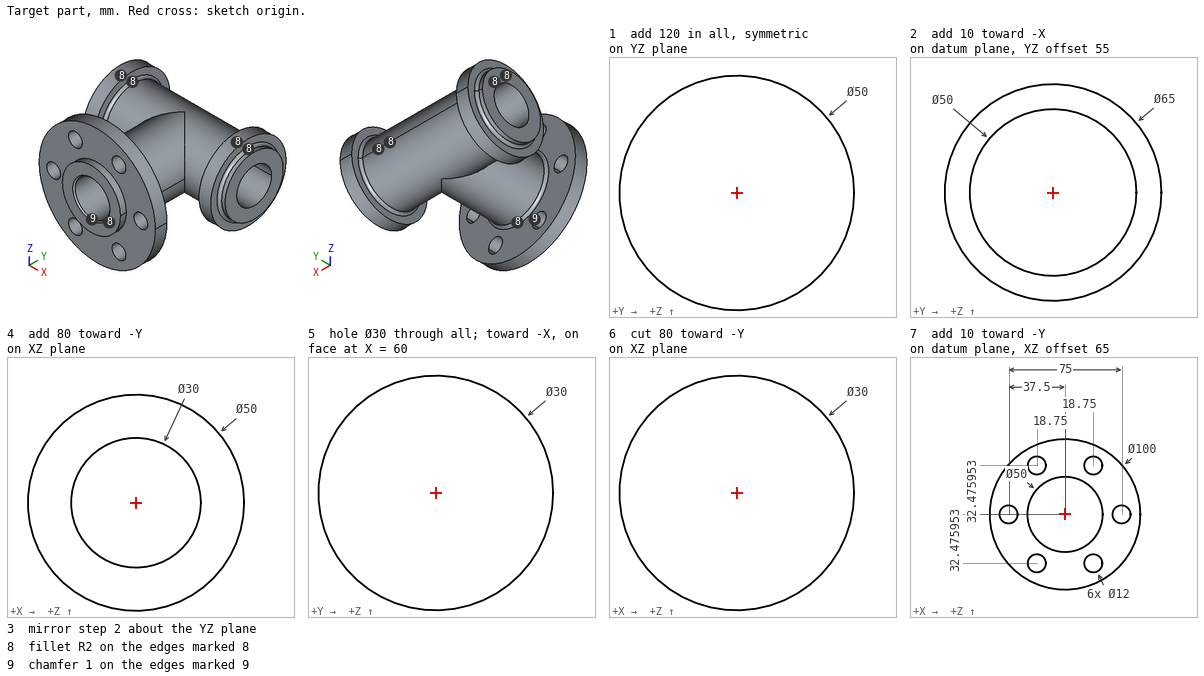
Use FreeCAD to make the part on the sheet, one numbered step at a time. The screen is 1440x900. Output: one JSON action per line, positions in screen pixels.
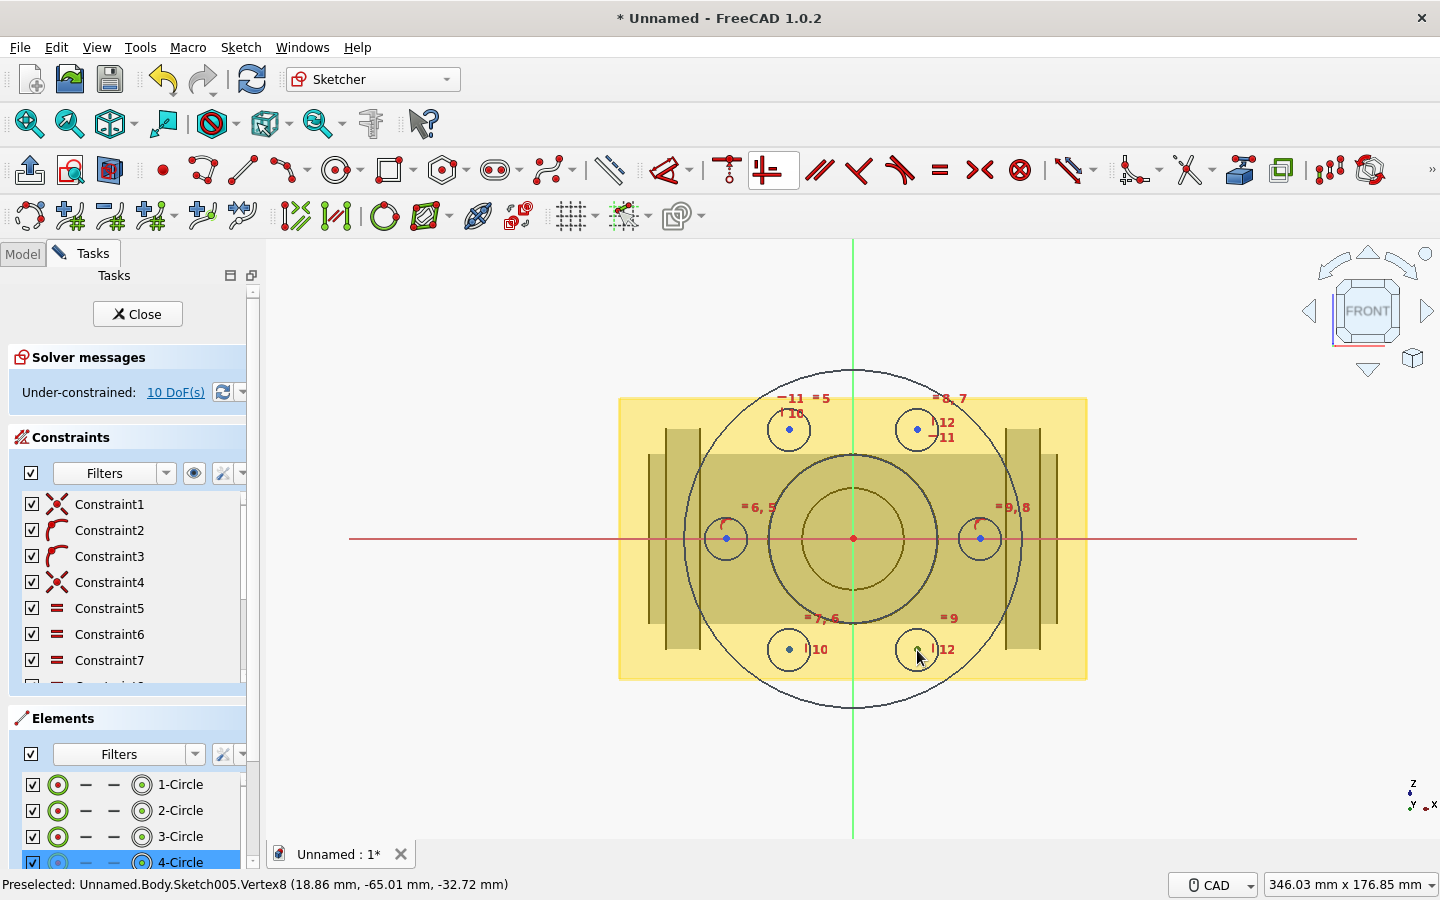
{"action": "key", "text": "h"}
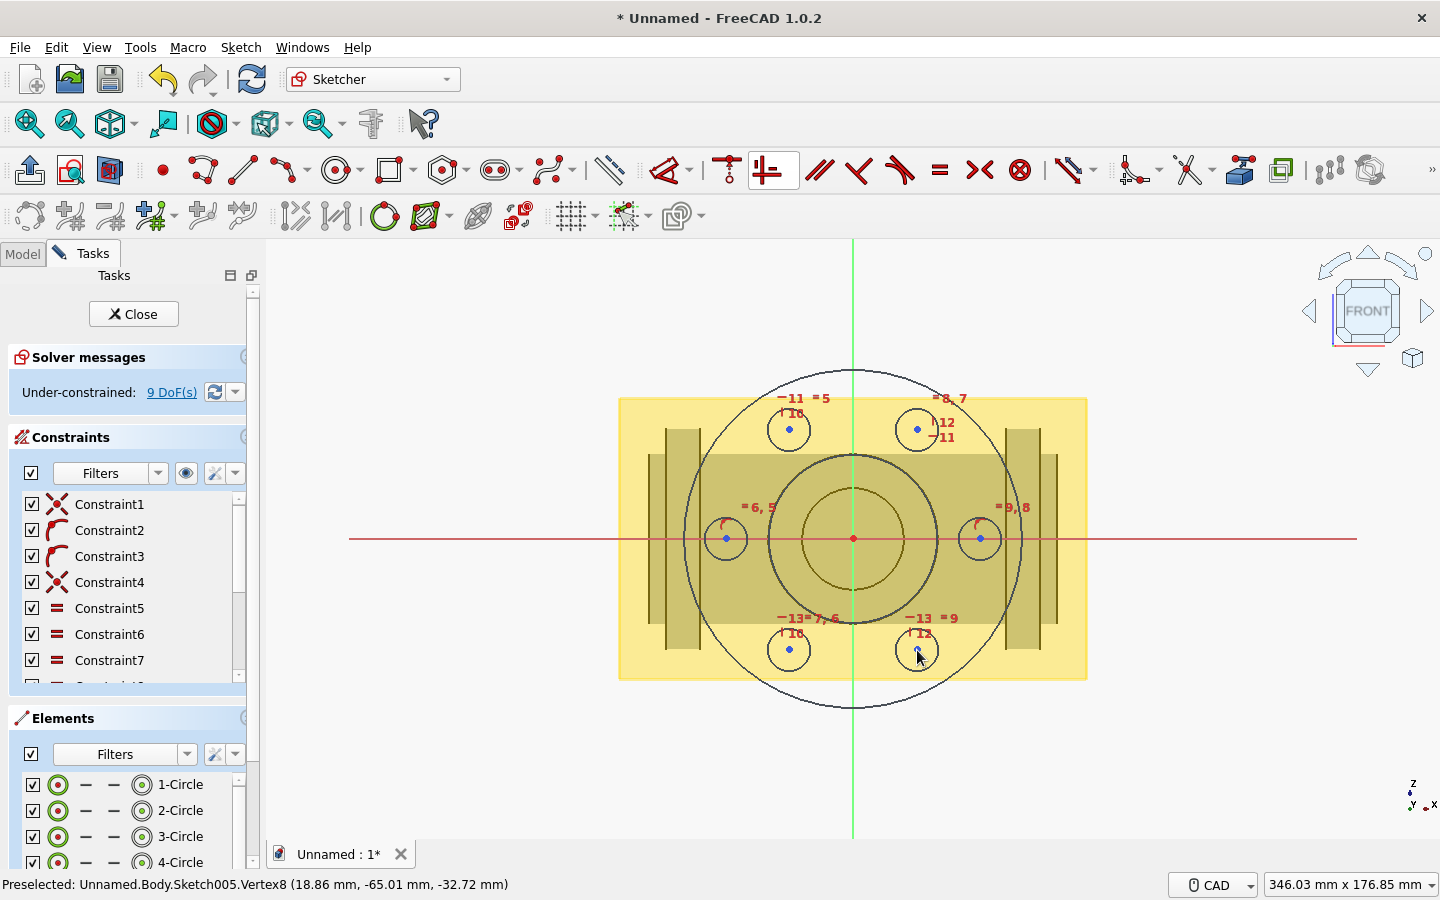
{"action": "left_click", "coordinate": [972, 419]}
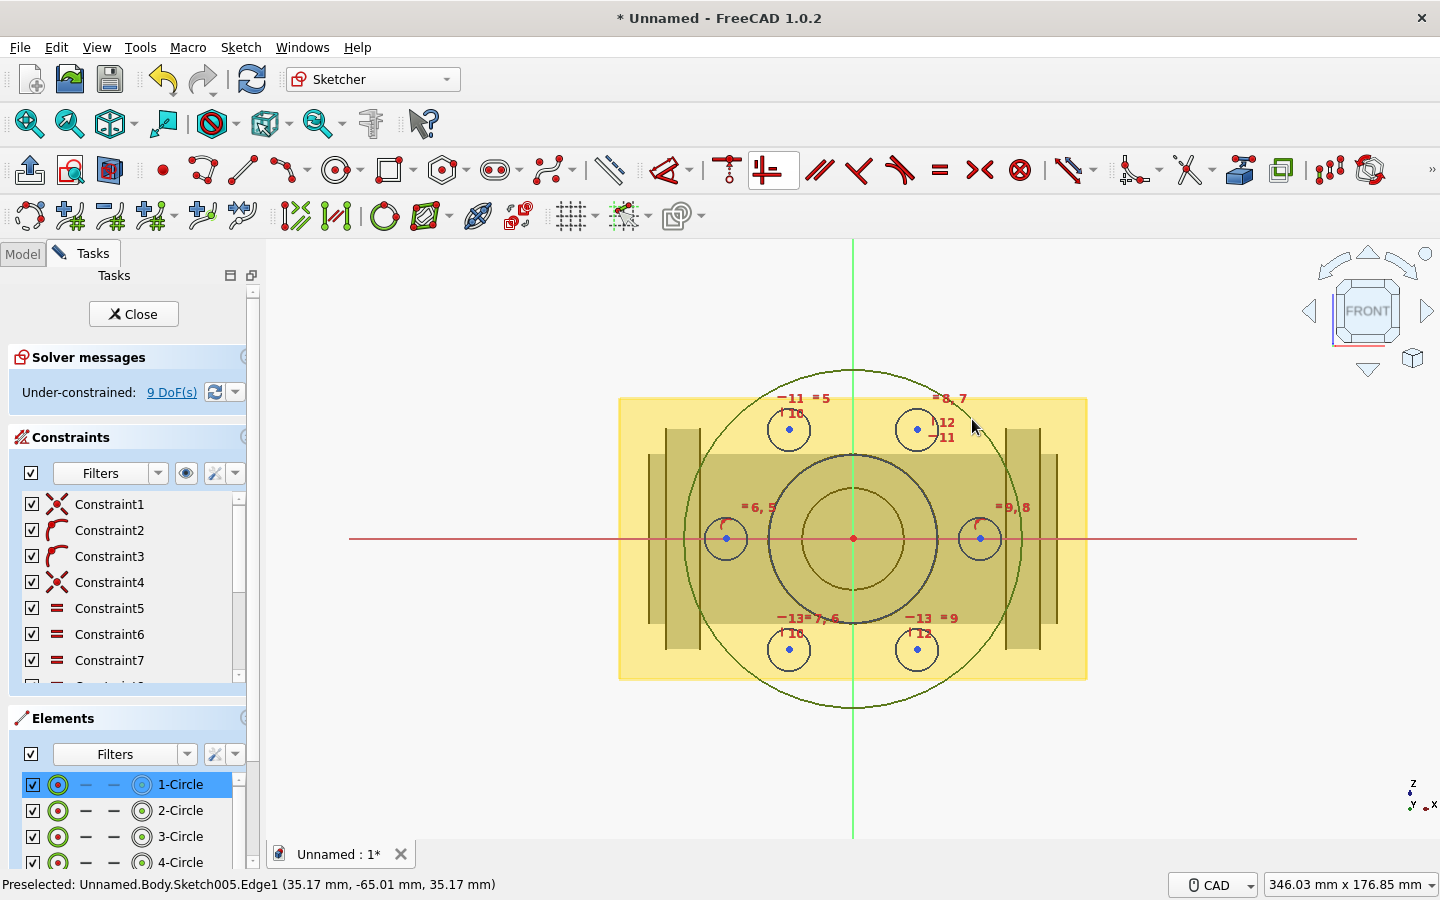
{"action": "key", "text": "k o"}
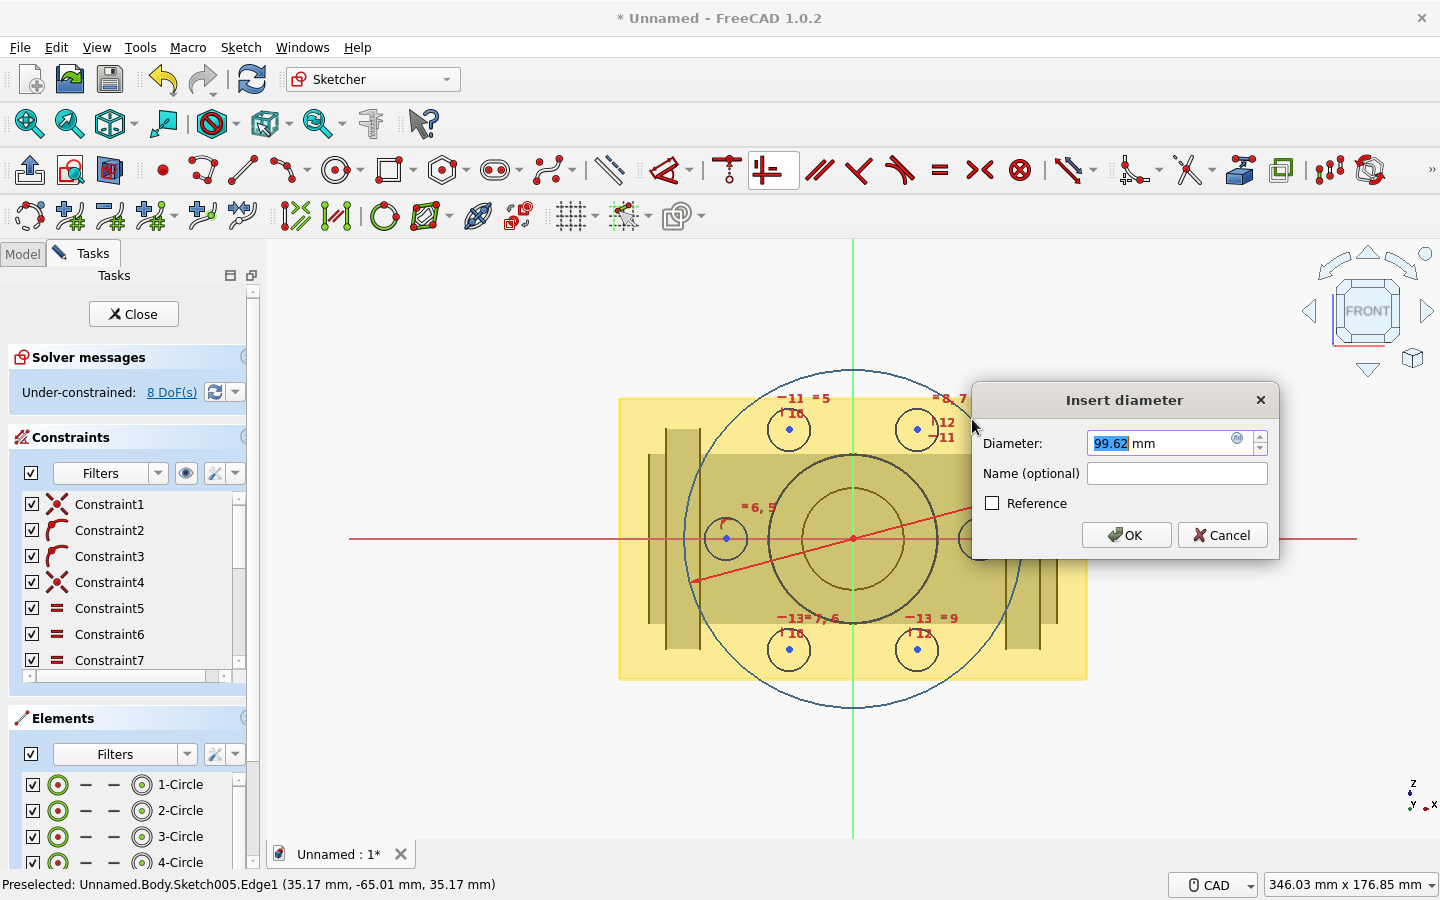
{"action": "type", "text": "100"}
{"action": "key", "text": "Return"}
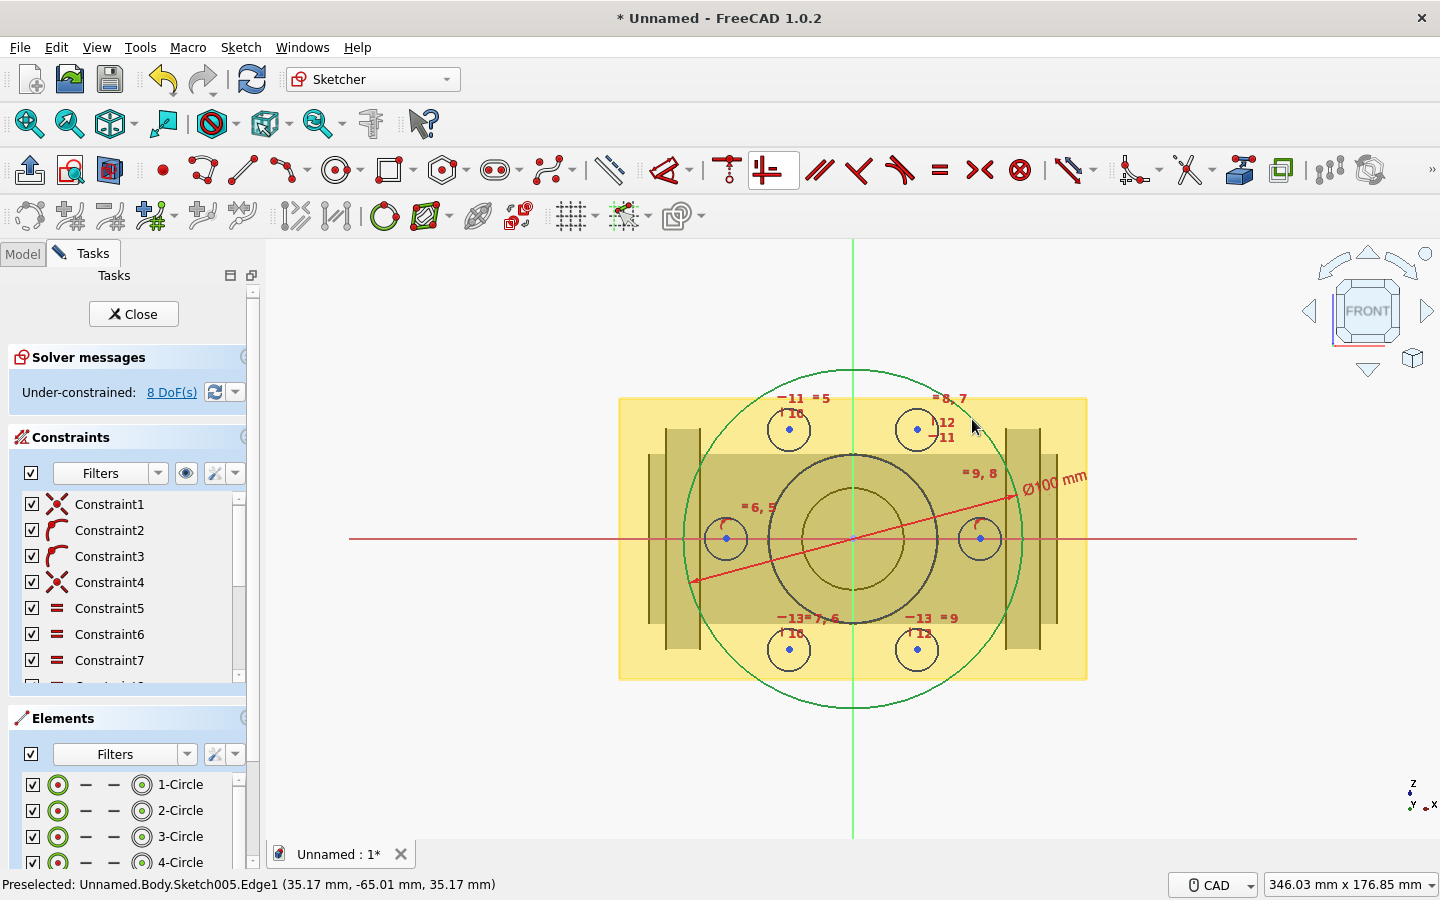
{"action": "left_click", "coordinate": [804, 415]}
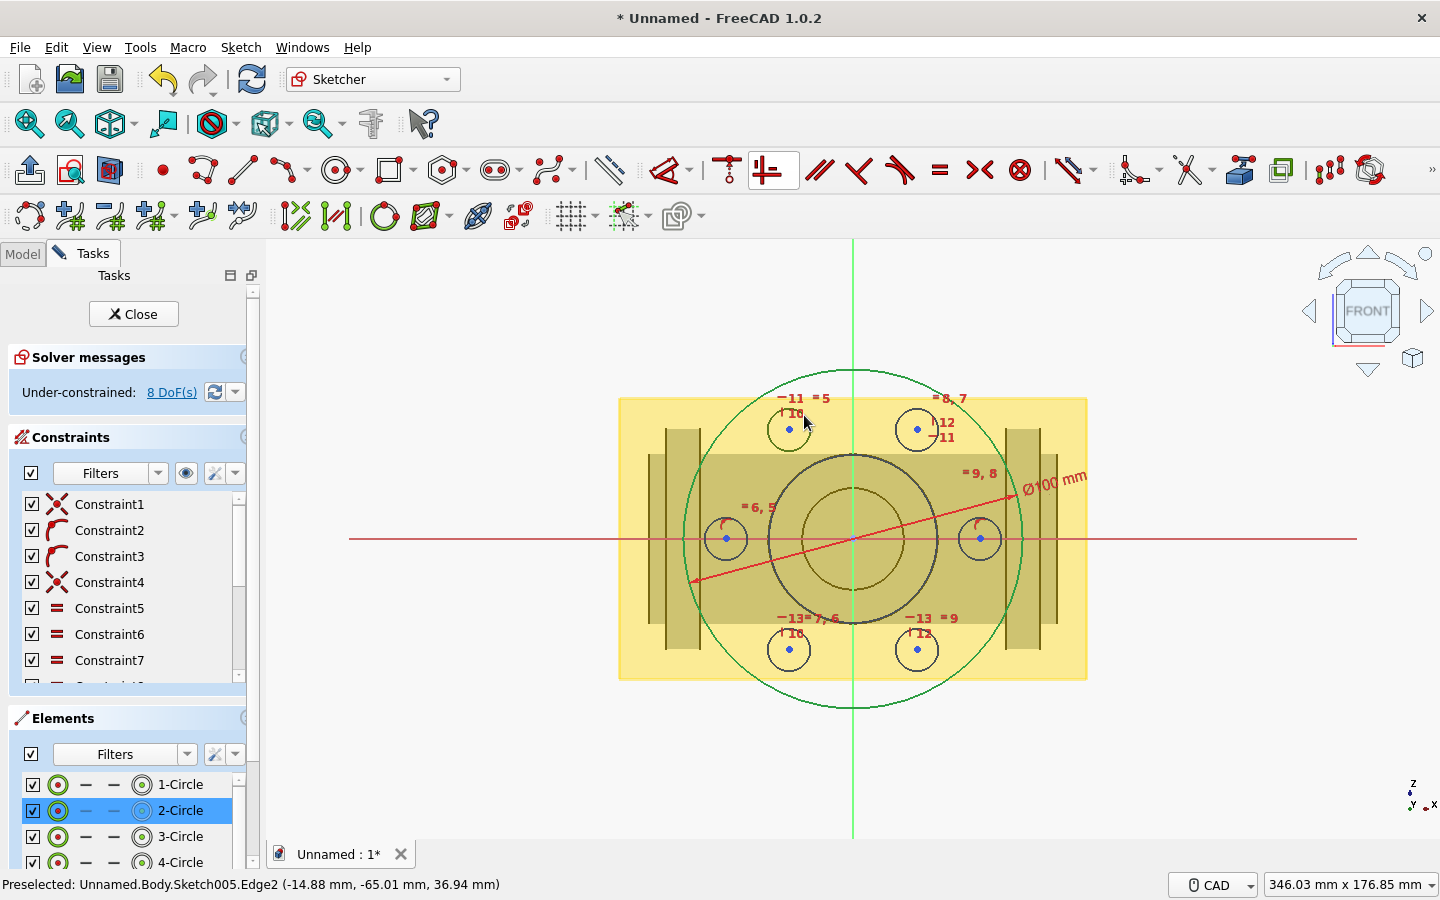
{"action": "key", "text": "k o"}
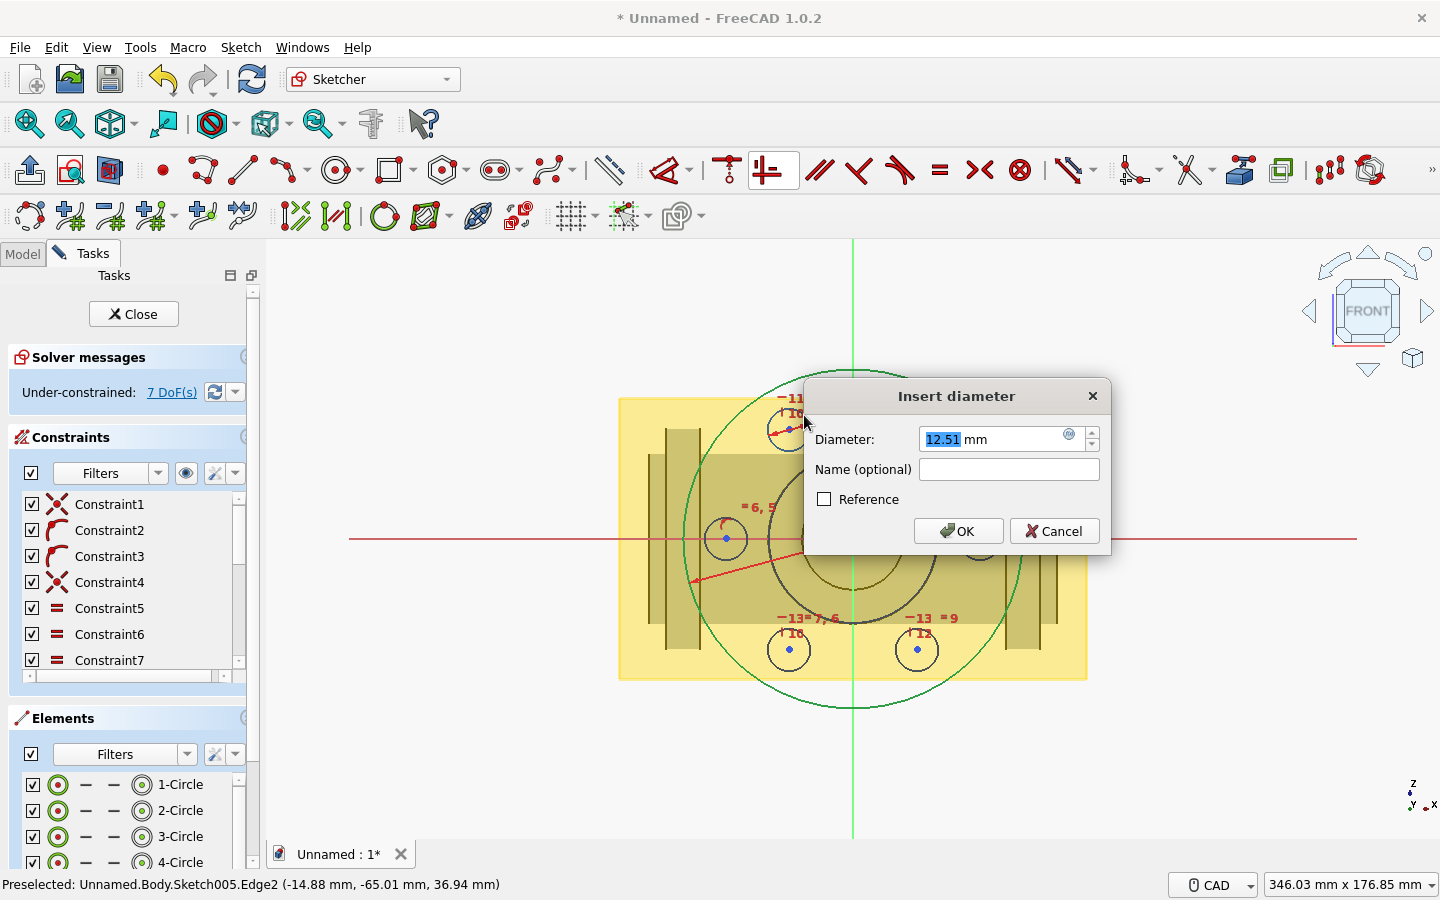
{"action": "type", "text": "12"}
{"action": "key", "text": "Return"}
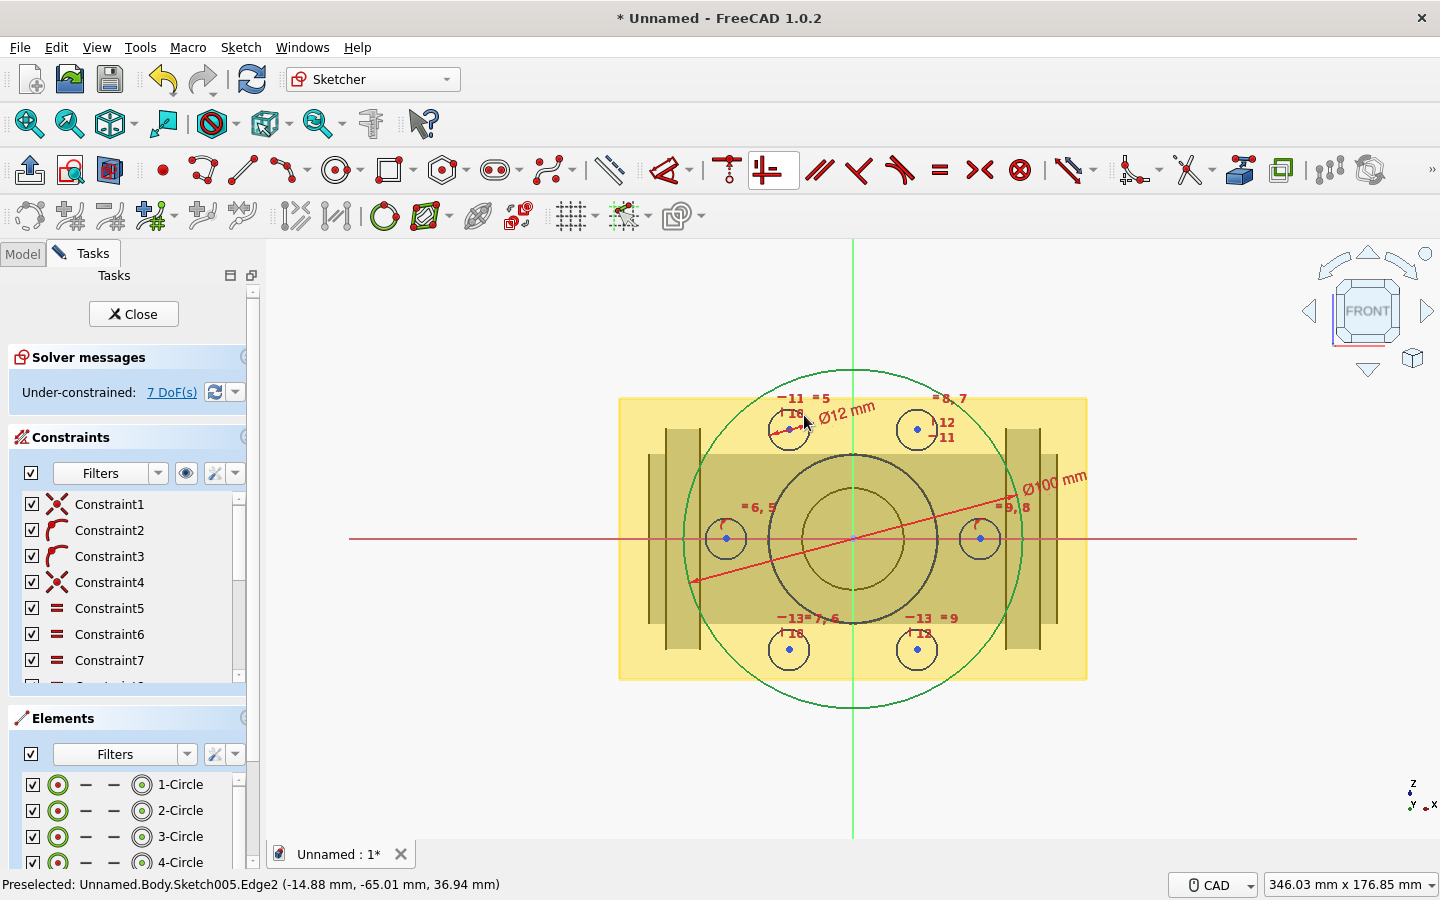
{"action": "left_click", "coordinate": [912, 479]}